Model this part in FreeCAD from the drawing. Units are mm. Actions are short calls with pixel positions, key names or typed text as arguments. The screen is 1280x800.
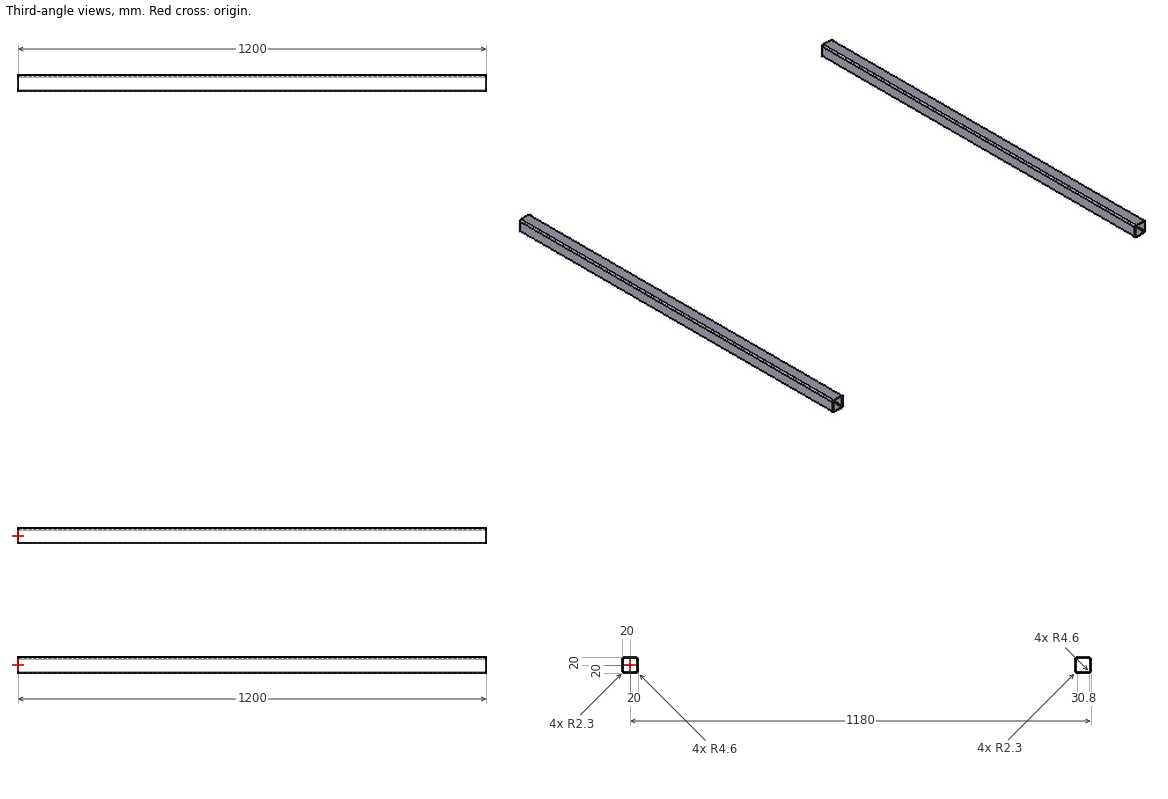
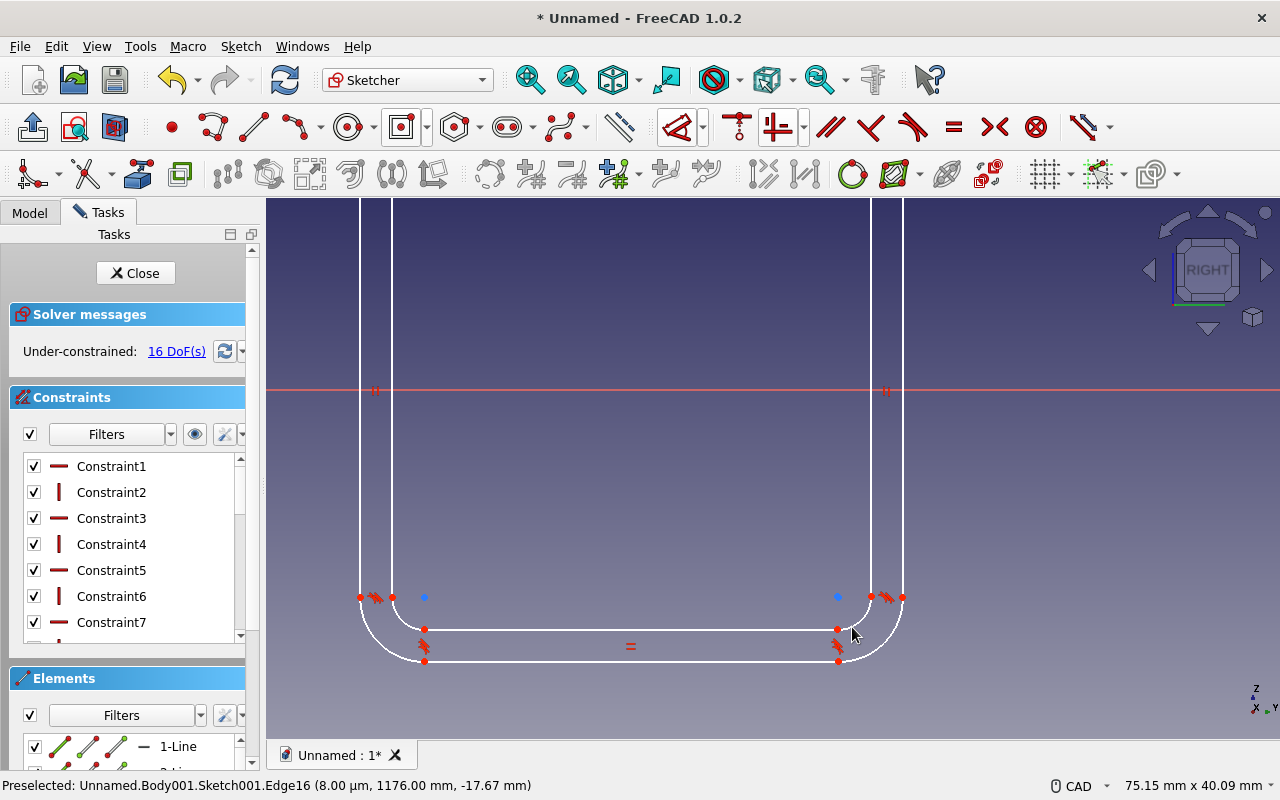
click(367, 627)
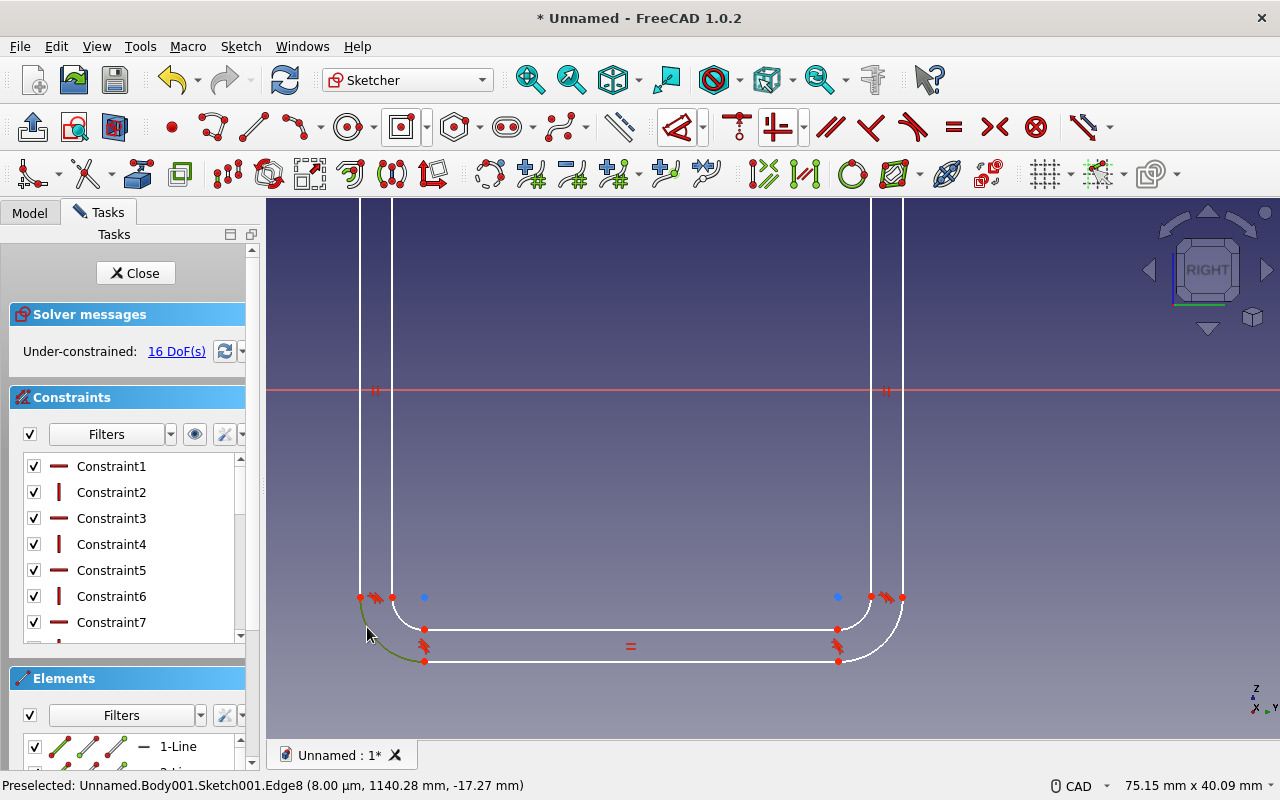
click(396, 612)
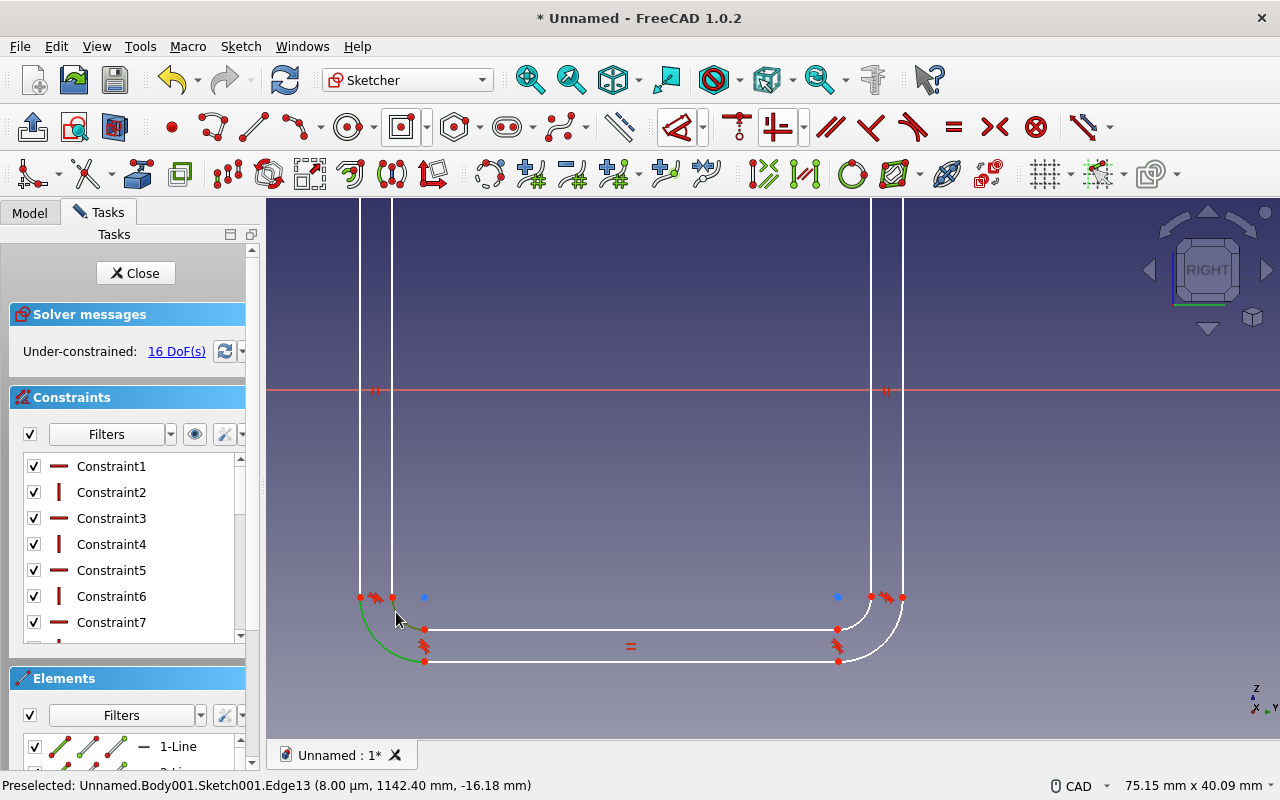
key(c)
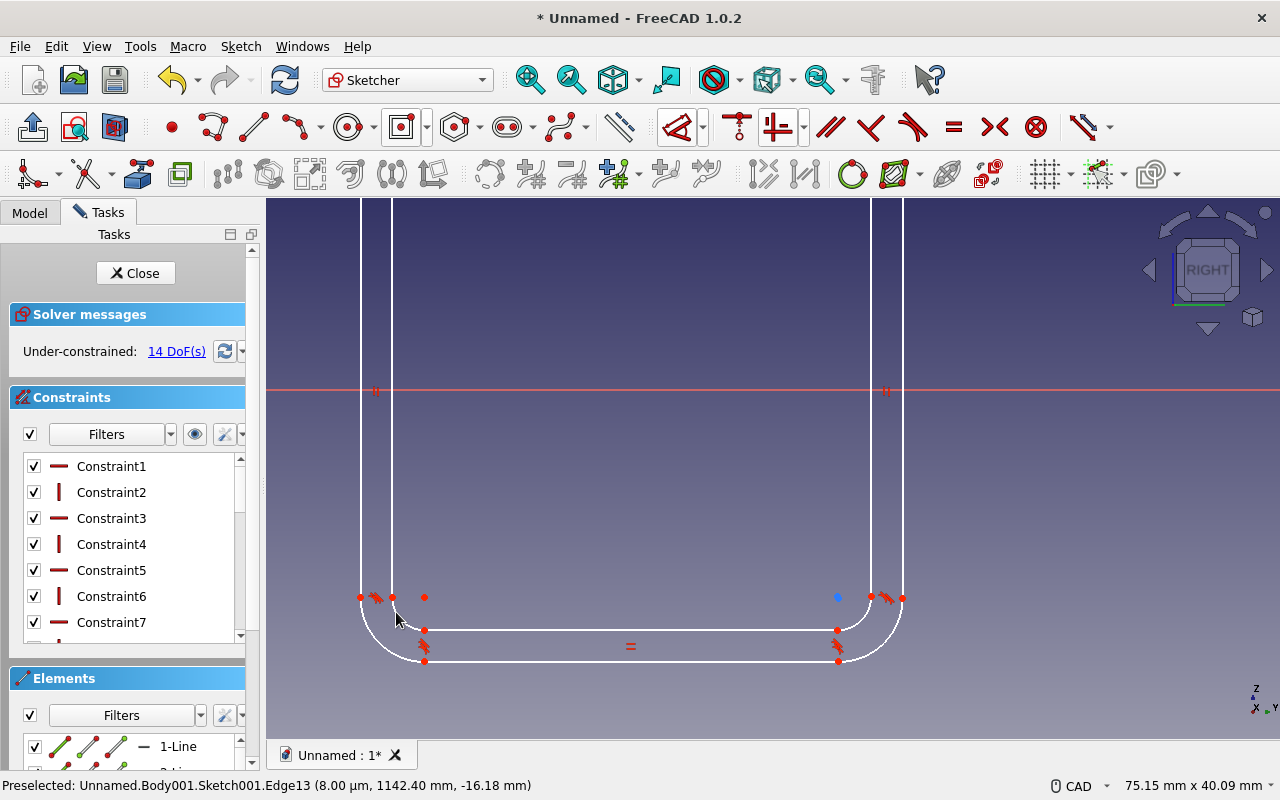
scroll(853, 628, down, 2)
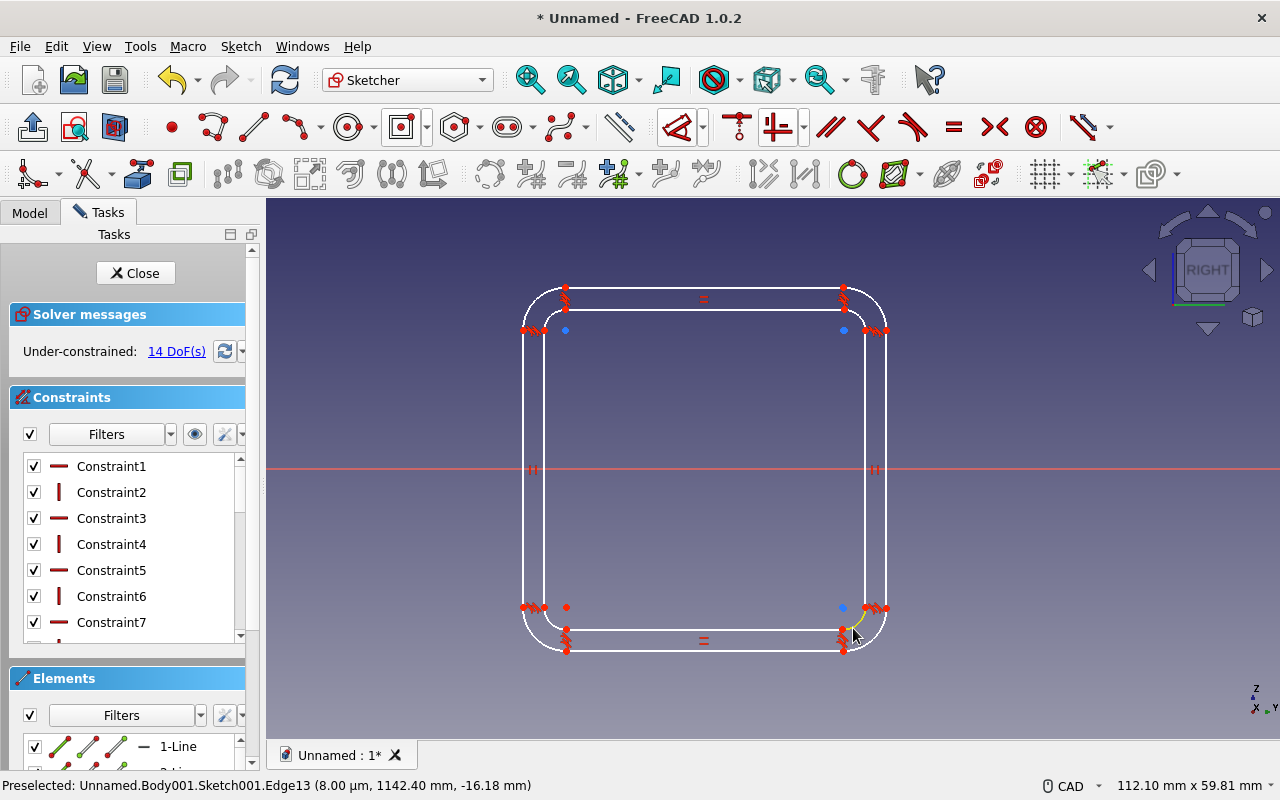
click(546, 292)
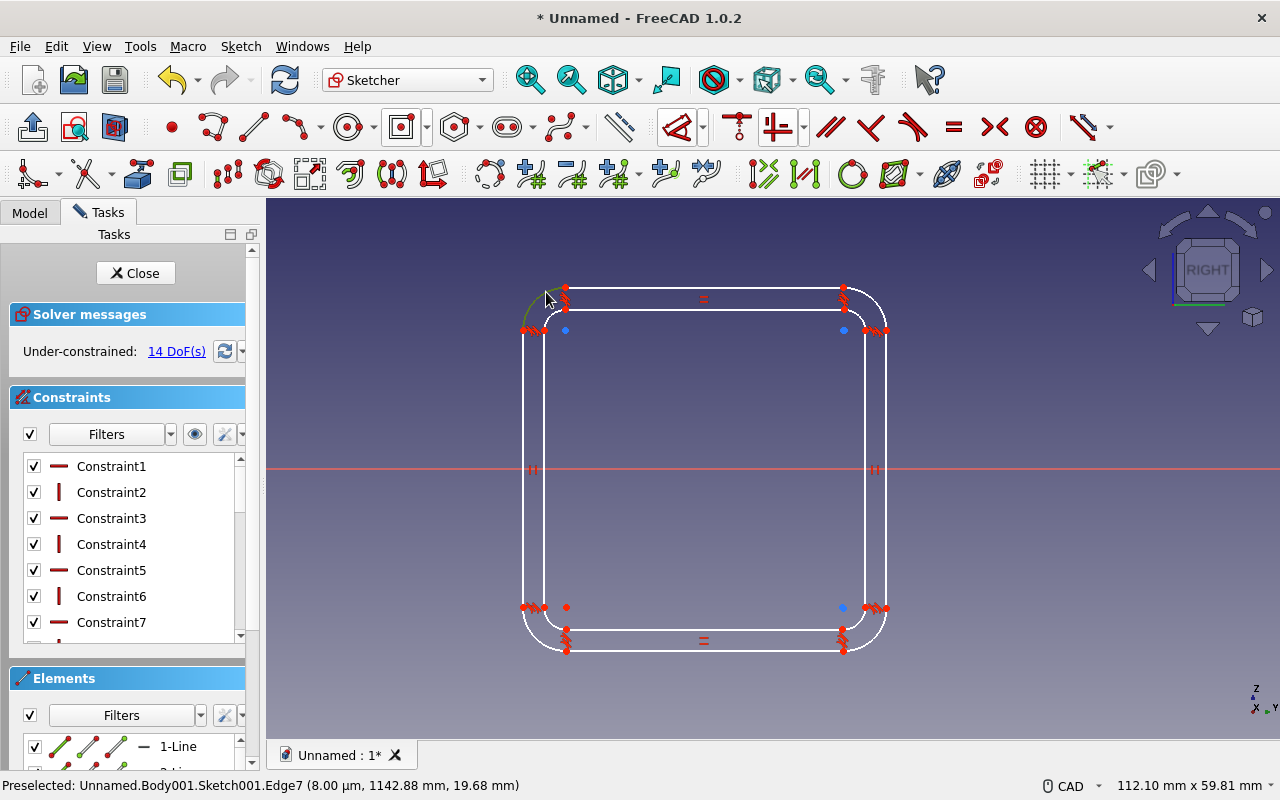
scroll(556, 312, up, 2)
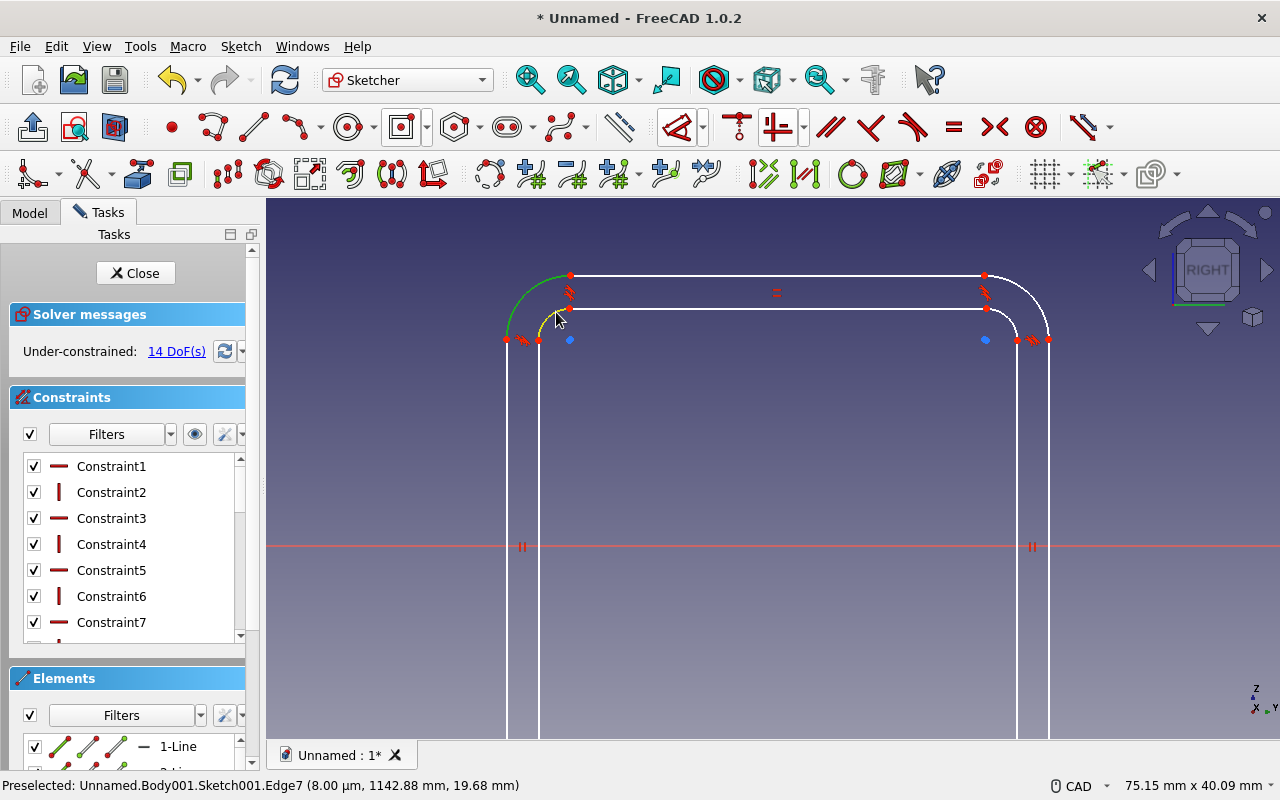
click(556, 312)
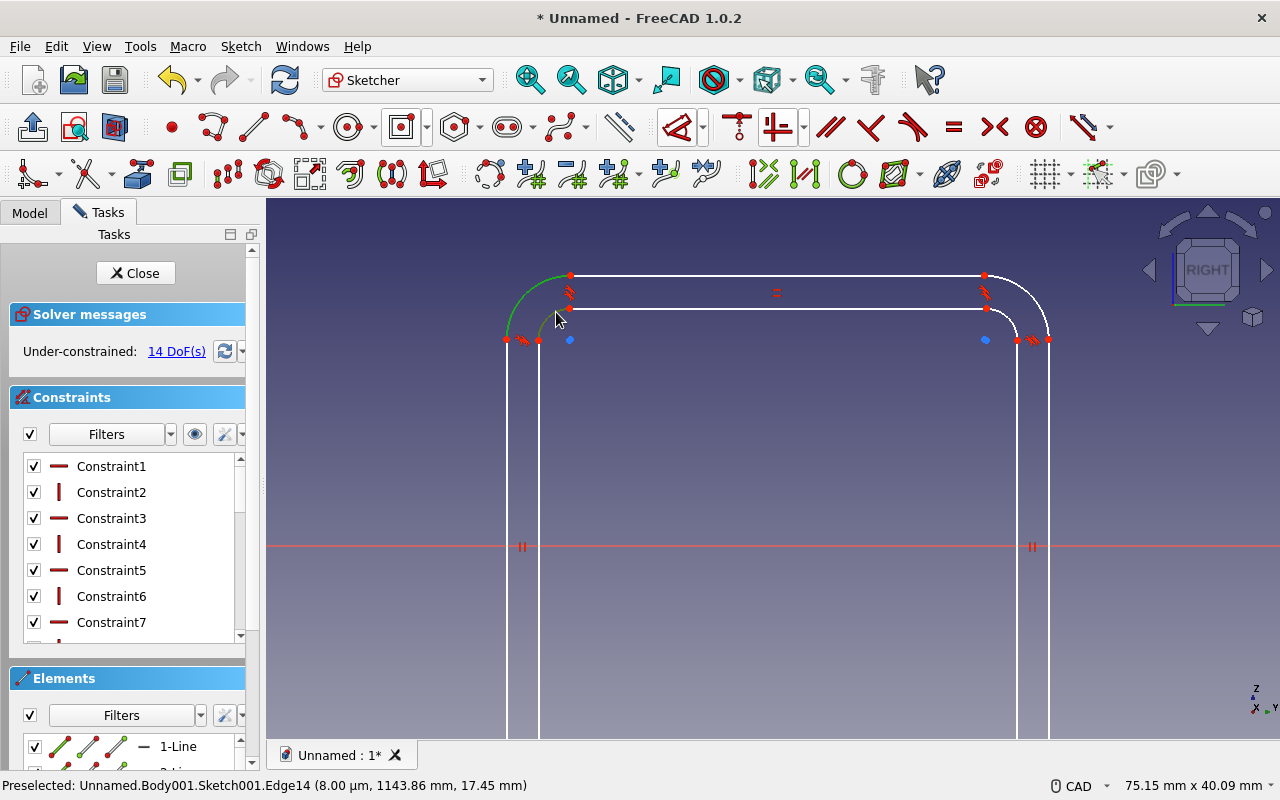
key(c)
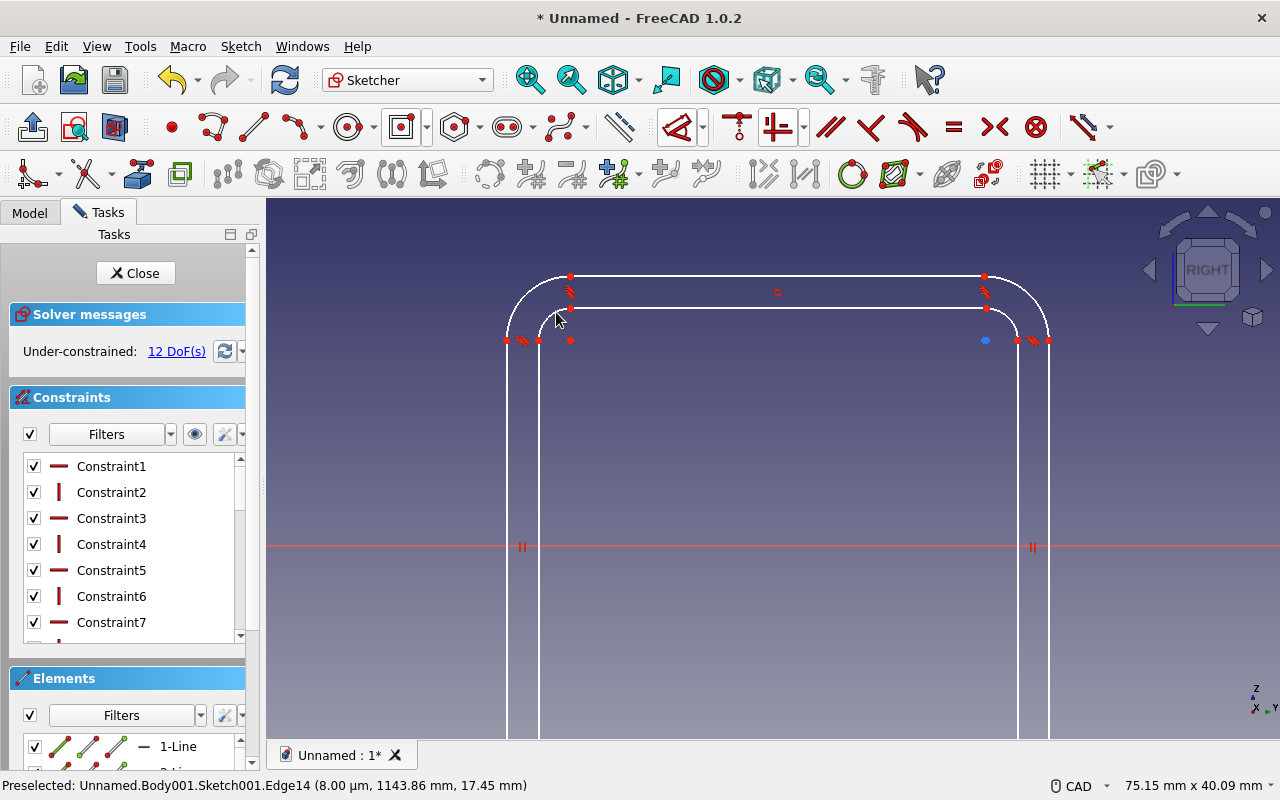
click(1042, 311)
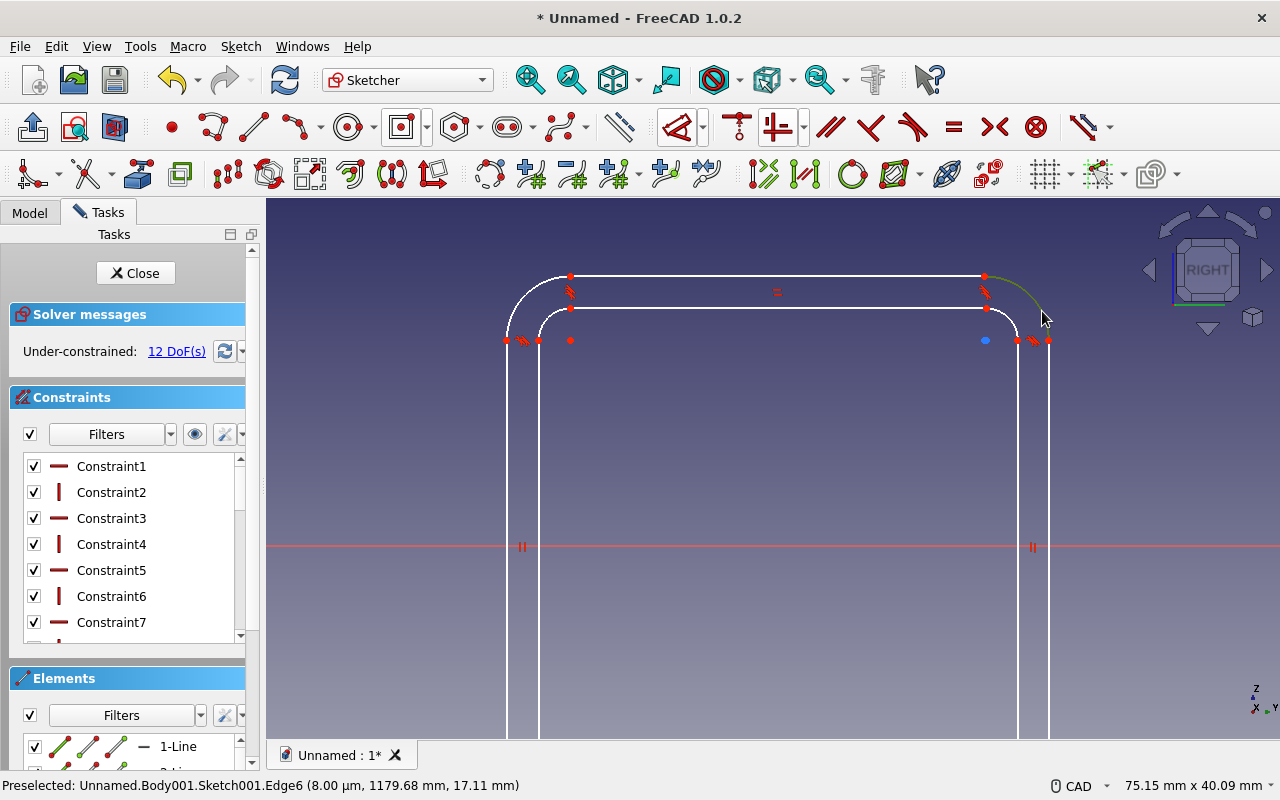
click(1014, 326)